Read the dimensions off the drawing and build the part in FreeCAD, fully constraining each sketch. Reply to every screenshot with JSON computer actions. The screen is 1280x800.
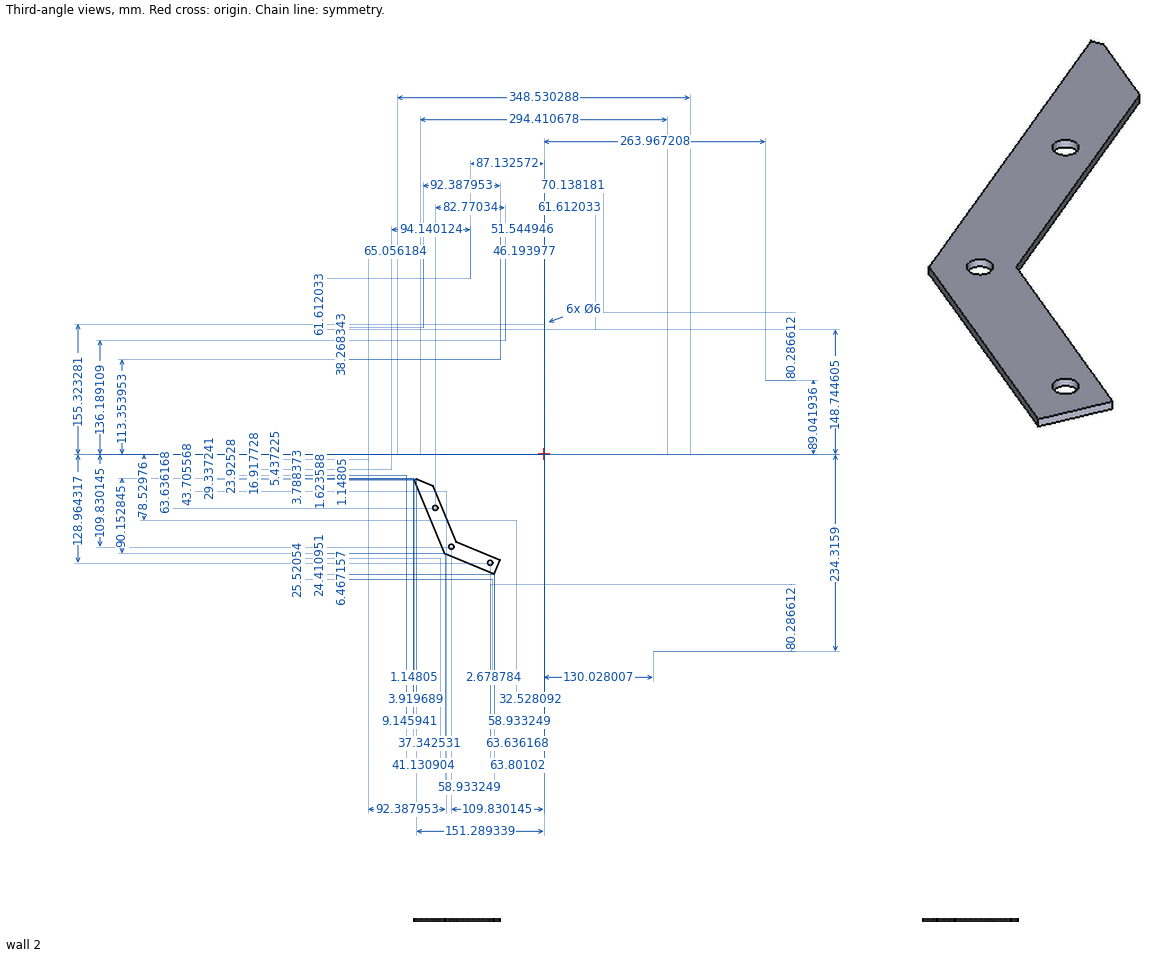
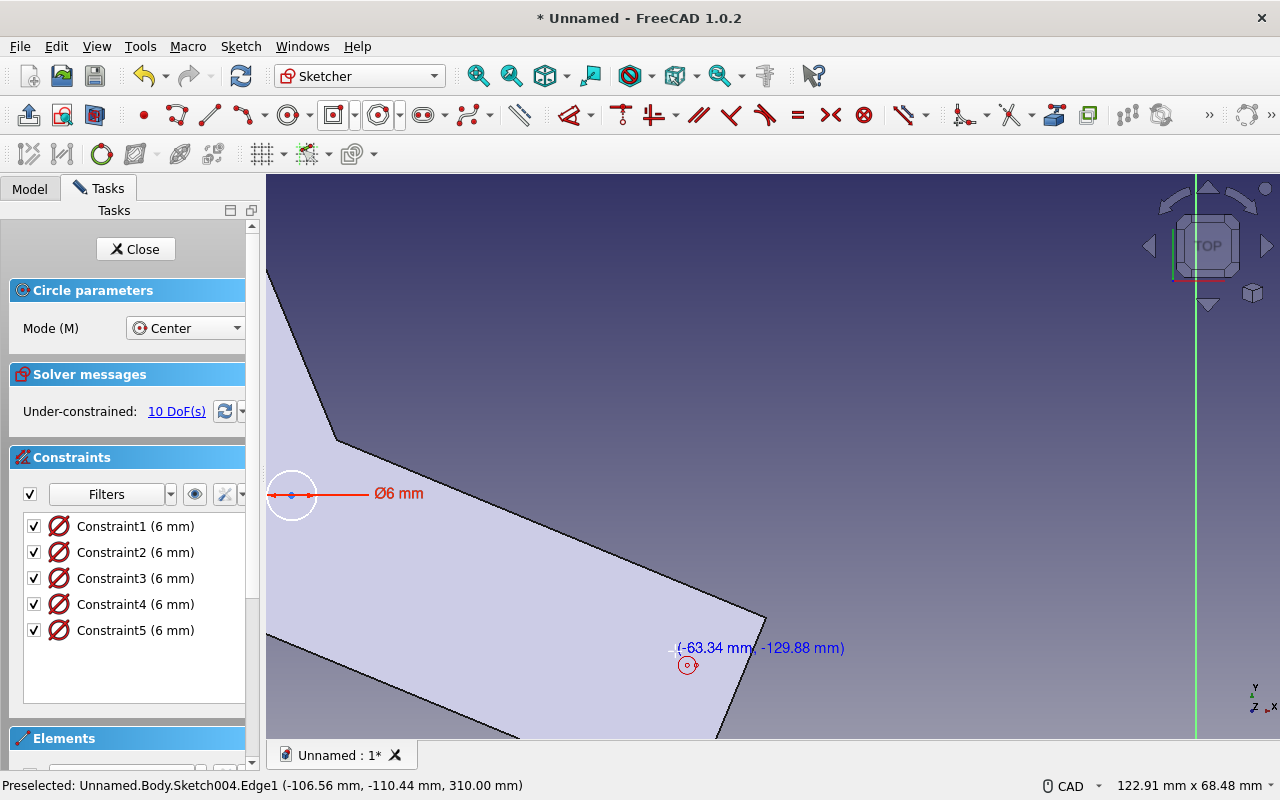
{"action": "scroll", "coordinate": [675, 651], "scroll_direction": "down", "scroll_amount": 9}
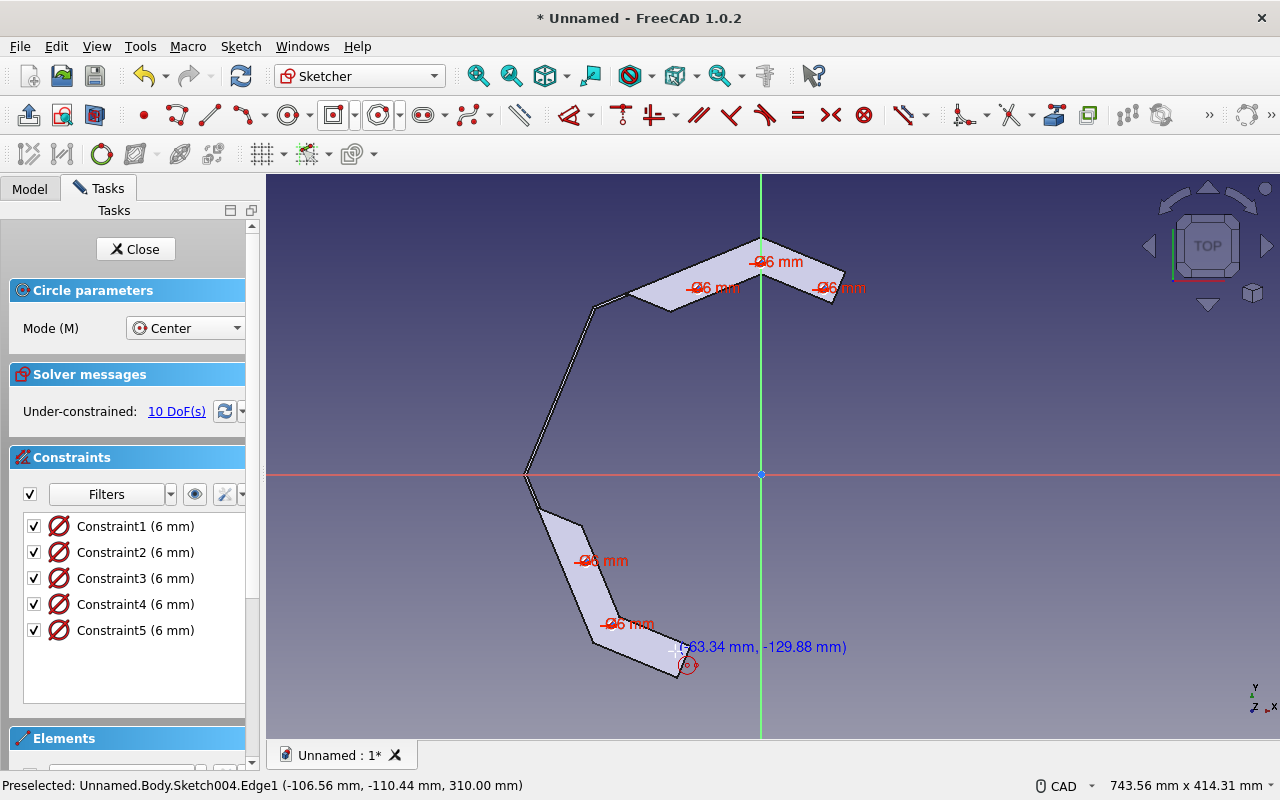
{"action": "left_click", "coordinate": [675, 651]}
{"action": "mouse_move", "coordinate": [677, 648]}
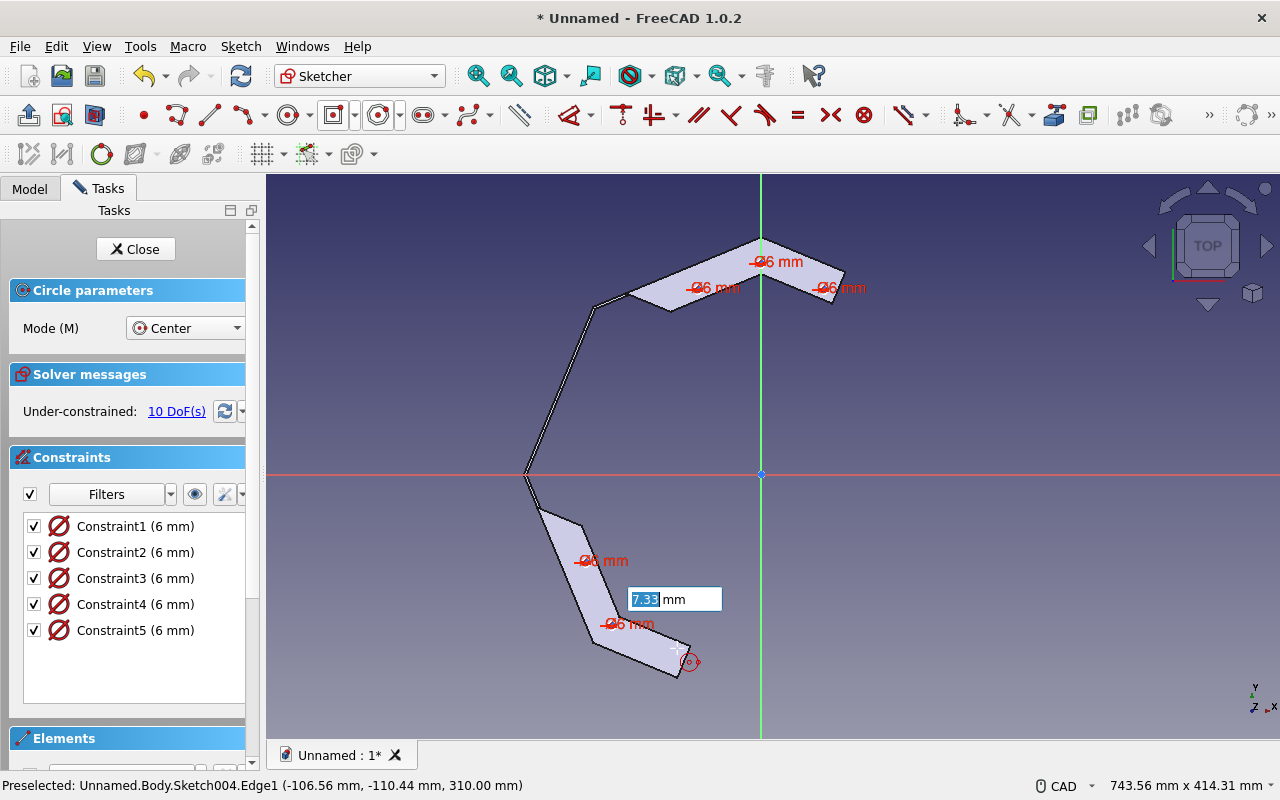
{"action": "type", "text": "6"}
{"action": "key", "text": "Return"}
{"action": "key", "text": "Escape"}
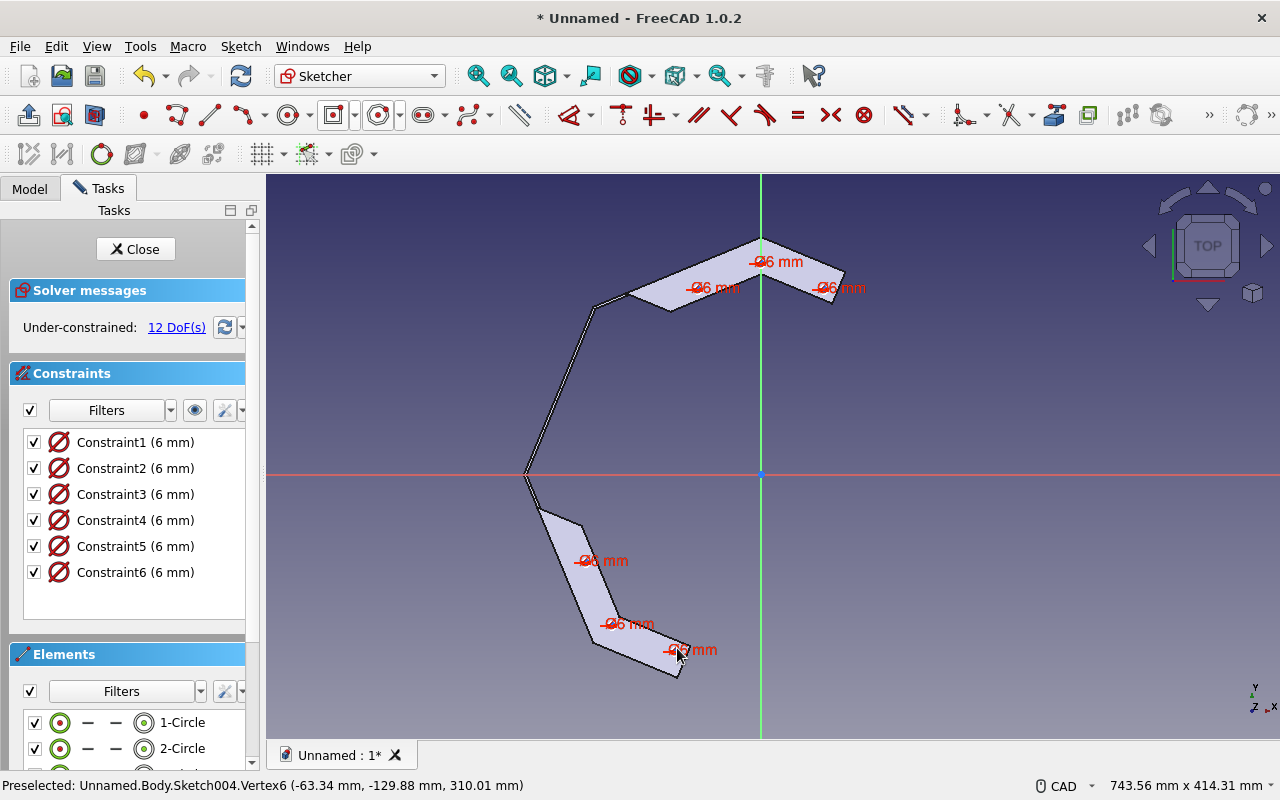
{"action": "left_click", "coordinate": [761, 264]}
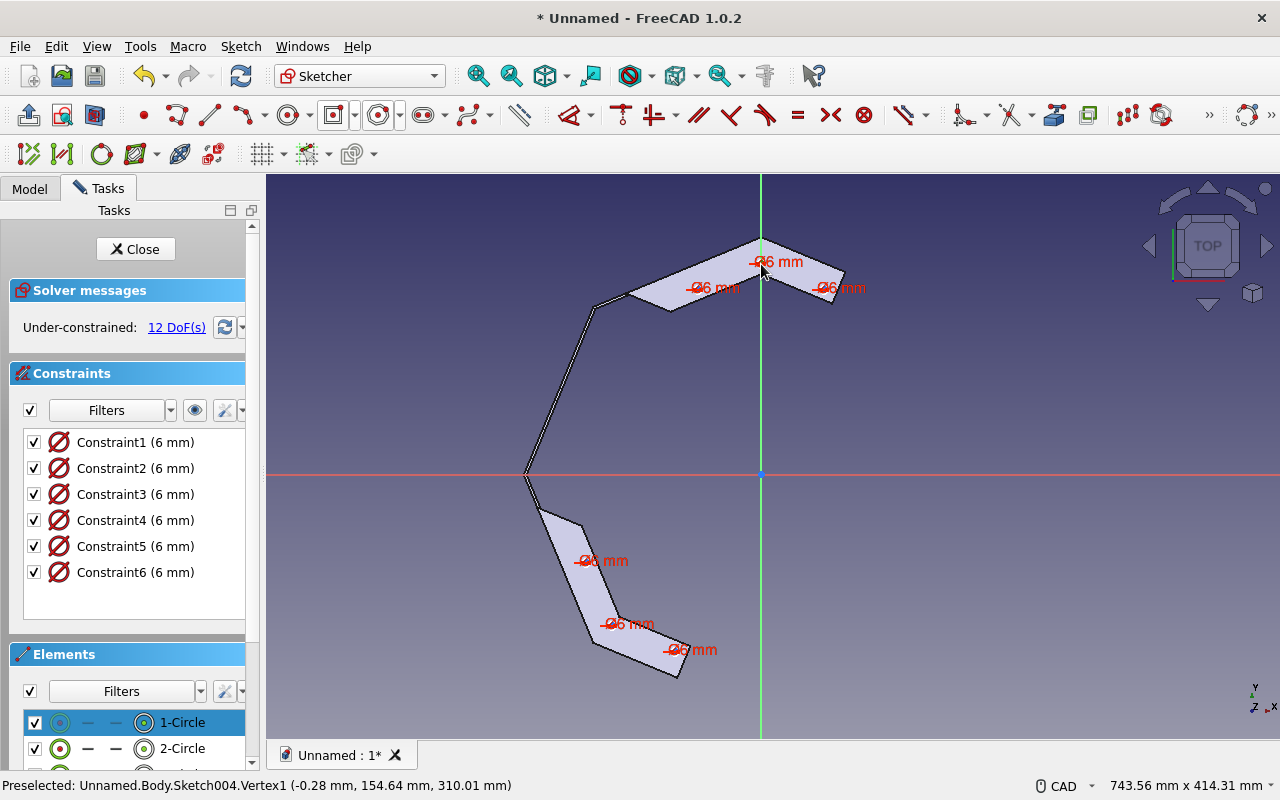
{"action": "left_click", "coordinate": [761, 675]}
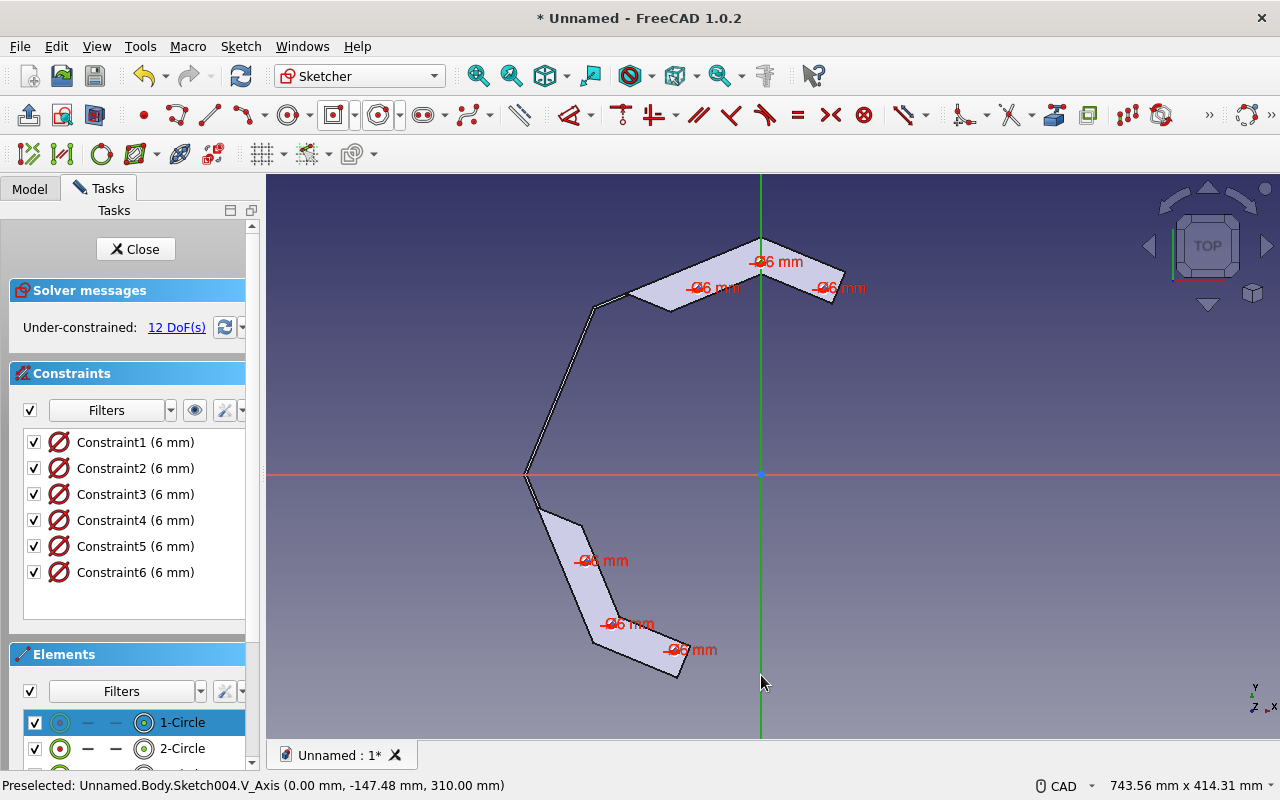
{"action": "left_click", "coordinate": [621, 116]}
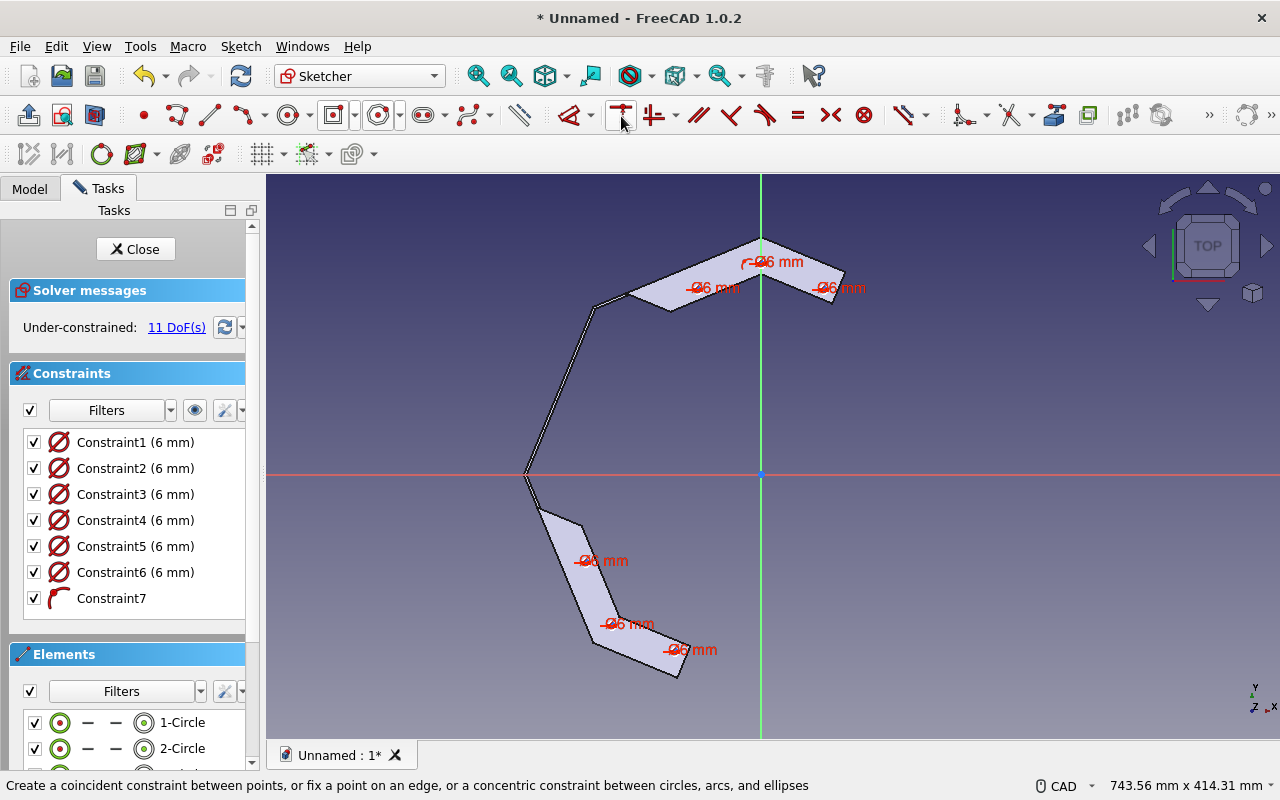
{"action": "left_click", "coordinate": [698, 290]}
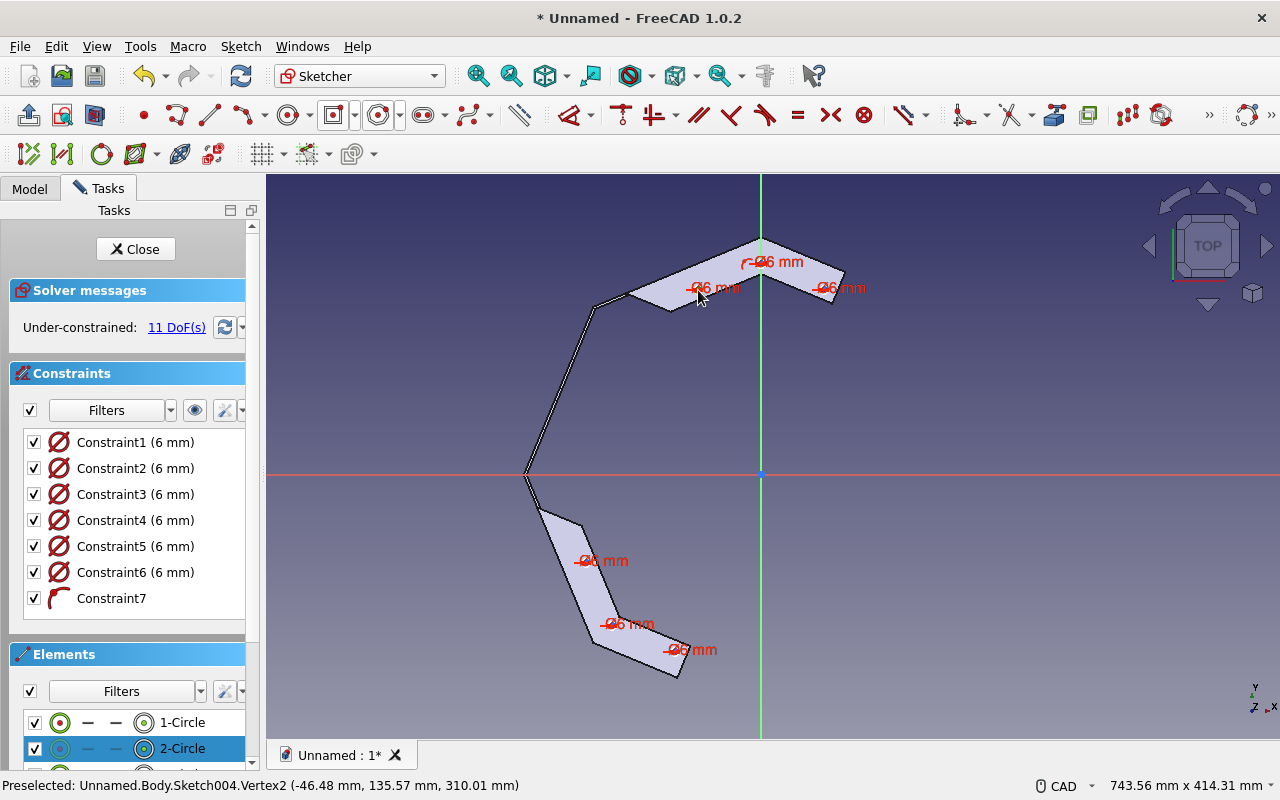
{"action": "left_click", "coordinate": [824, 290]}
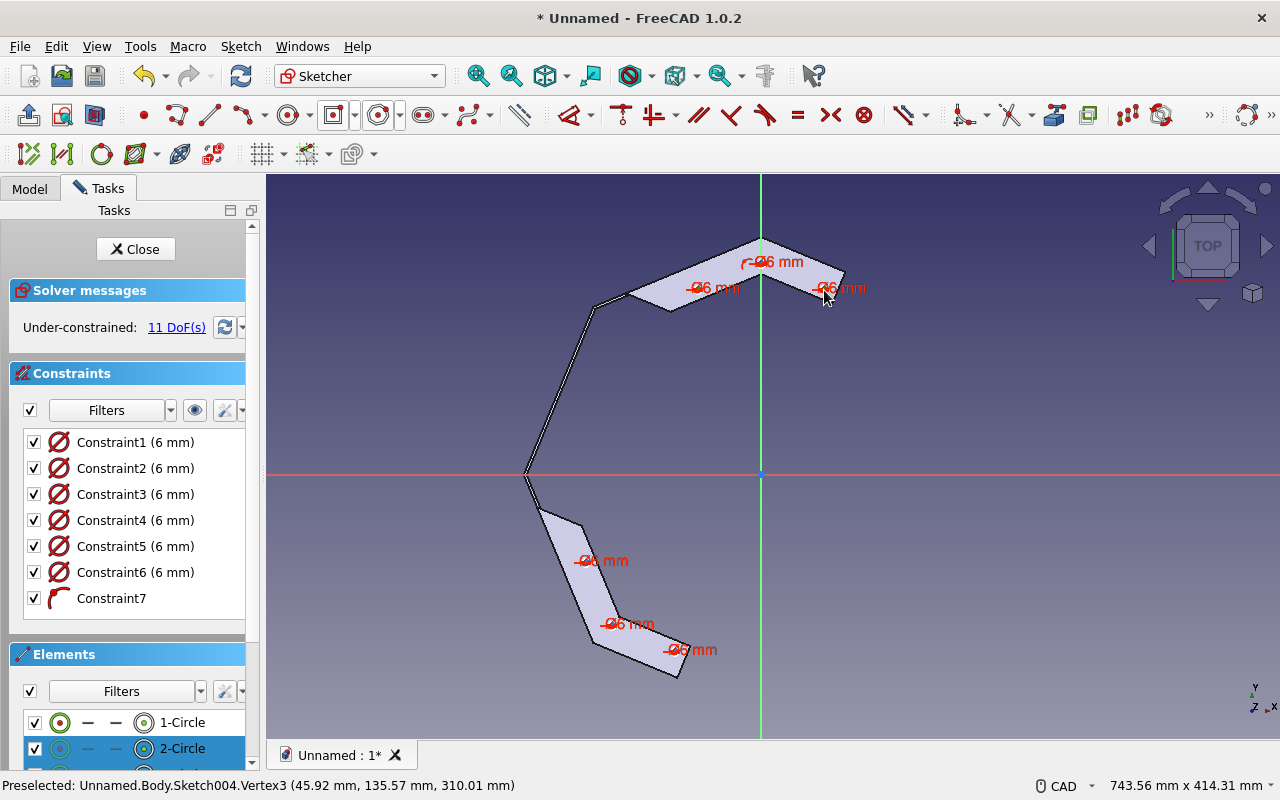
{"action": "left_click", "coordinate": [761, 675]}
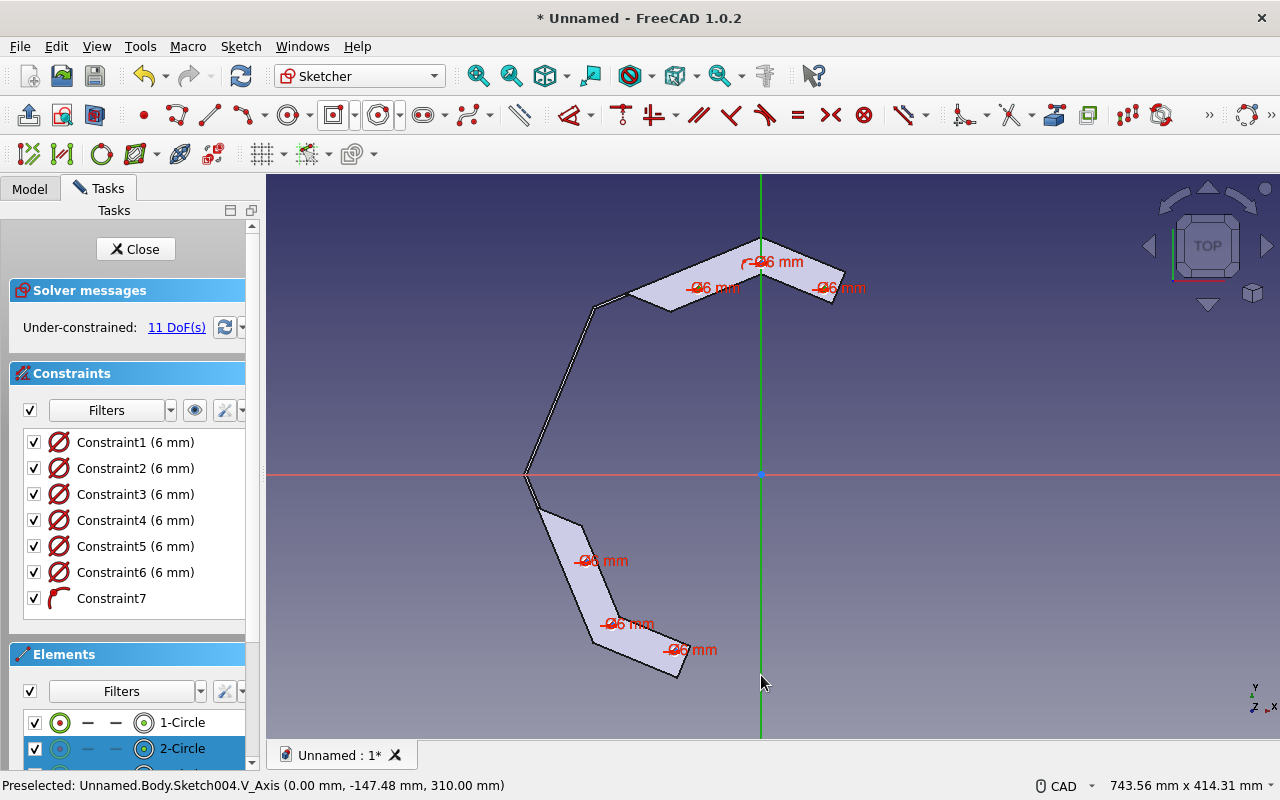
{"action": "left_click", "coordinate": [831, 116]}